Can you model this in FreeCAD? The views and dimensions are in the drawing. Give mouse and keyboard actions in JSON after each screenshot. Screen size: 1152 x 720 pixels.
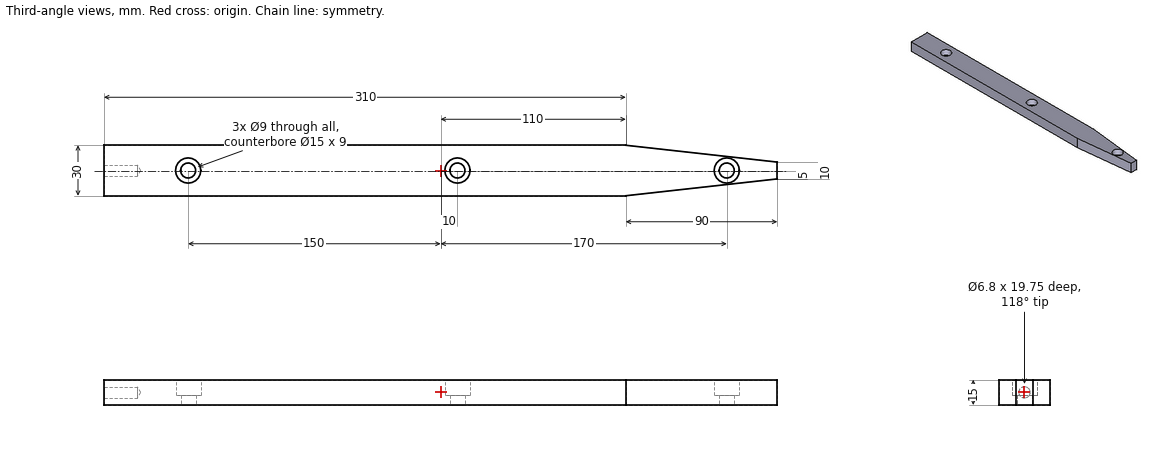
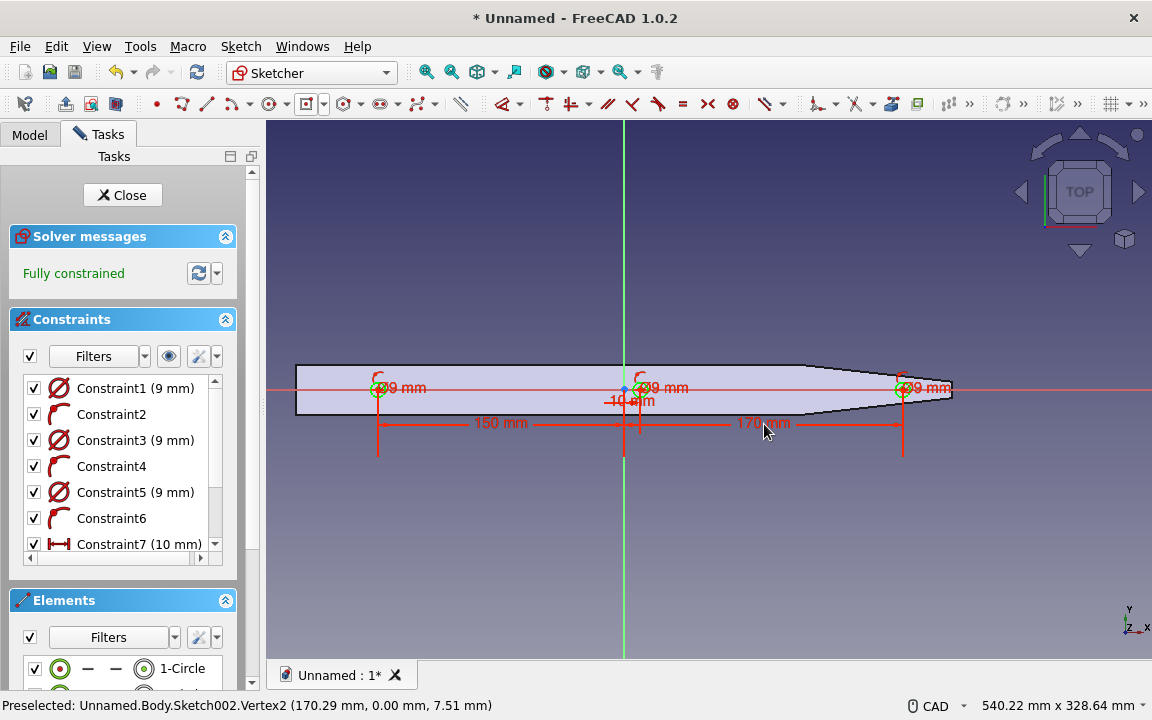
{"action": "left_click", "coordinate": [123, 195]}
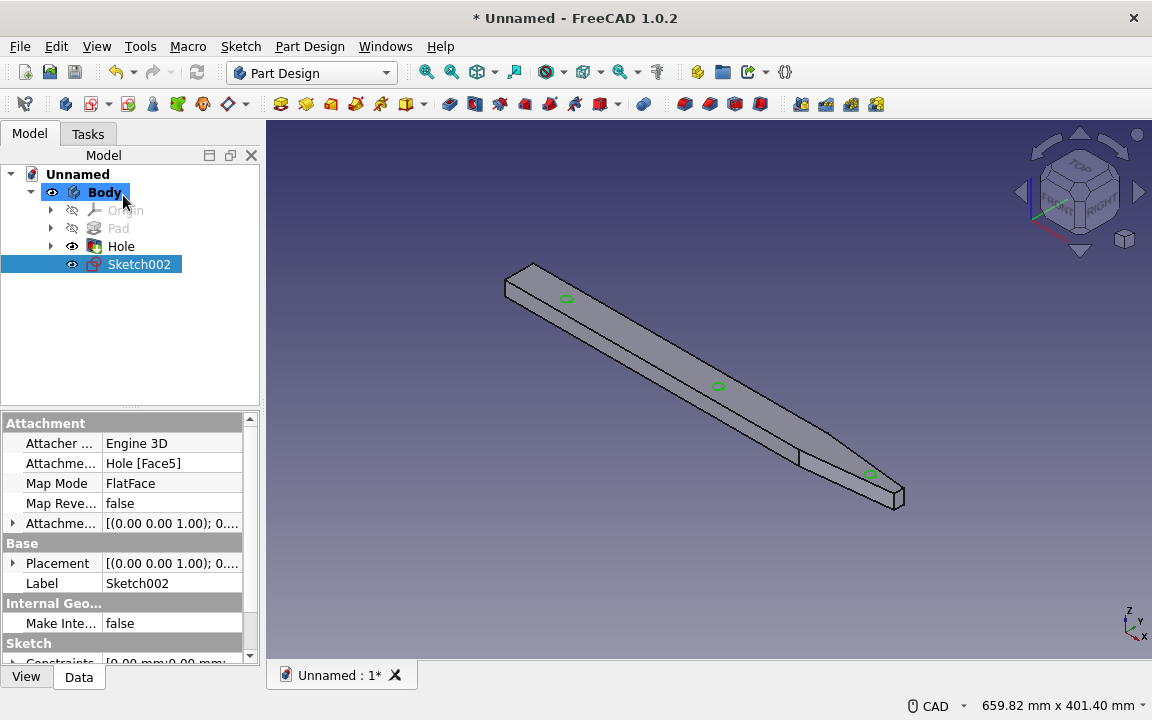
{"action": "left_click", "coordinate": [475, 104]}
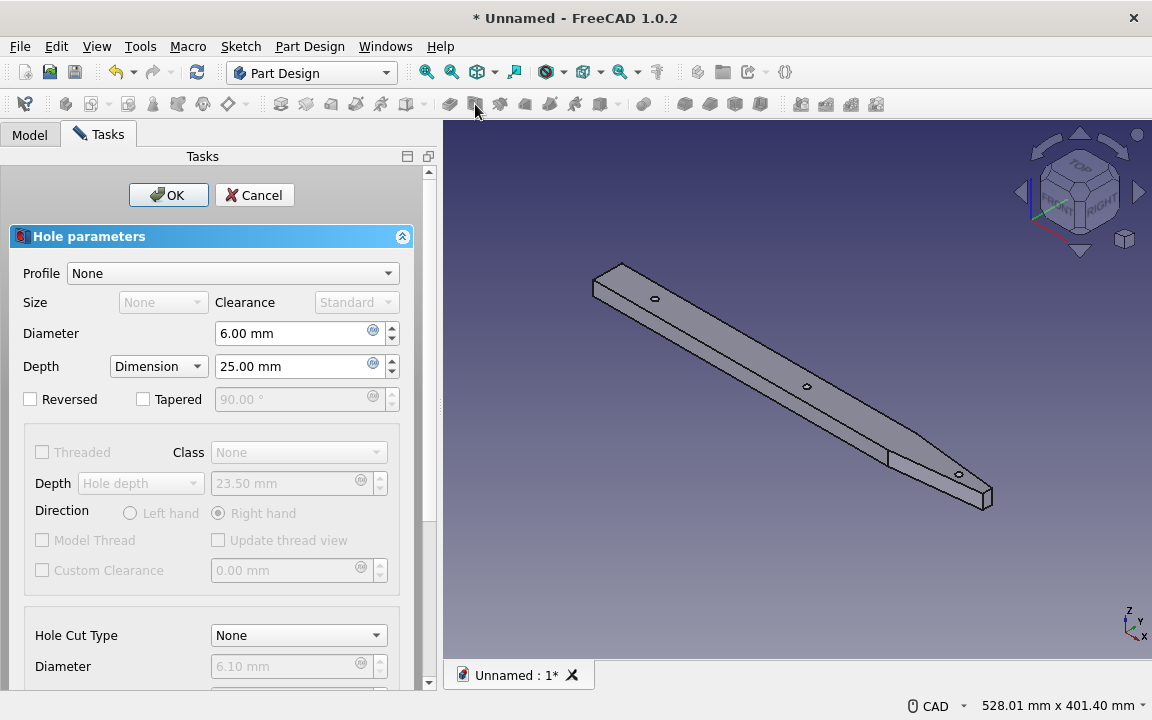
{"action": "triple_click", "coordinate": [300, 334]}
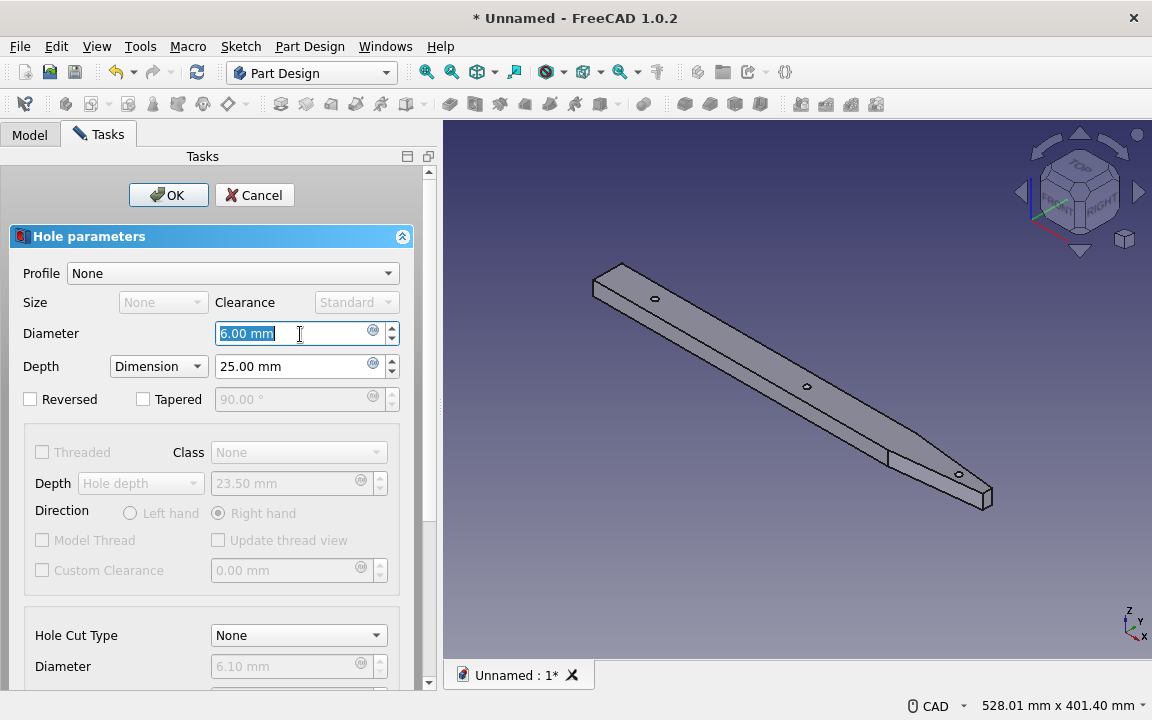
{"action": "type", "text": "9"}
{"action": "key", "text": "Tab"}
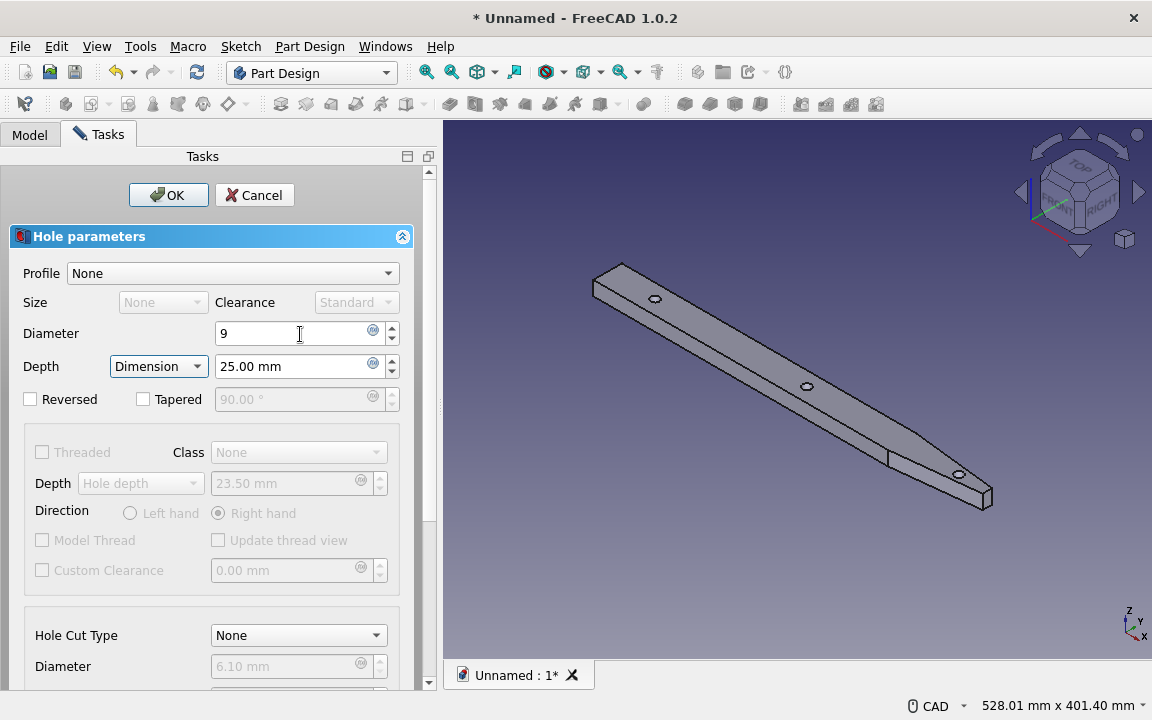
{"action": "left_click", "coordinate": [160, 366]}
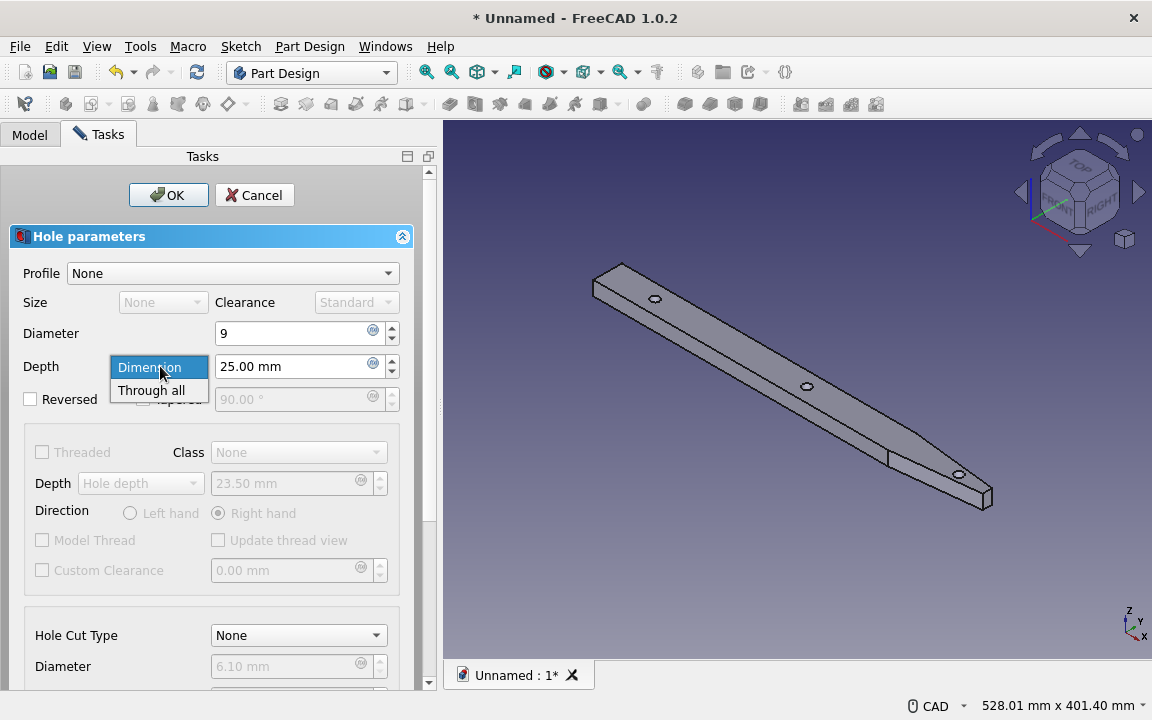
{"action": "left_click", "coordinate": [158, 390]}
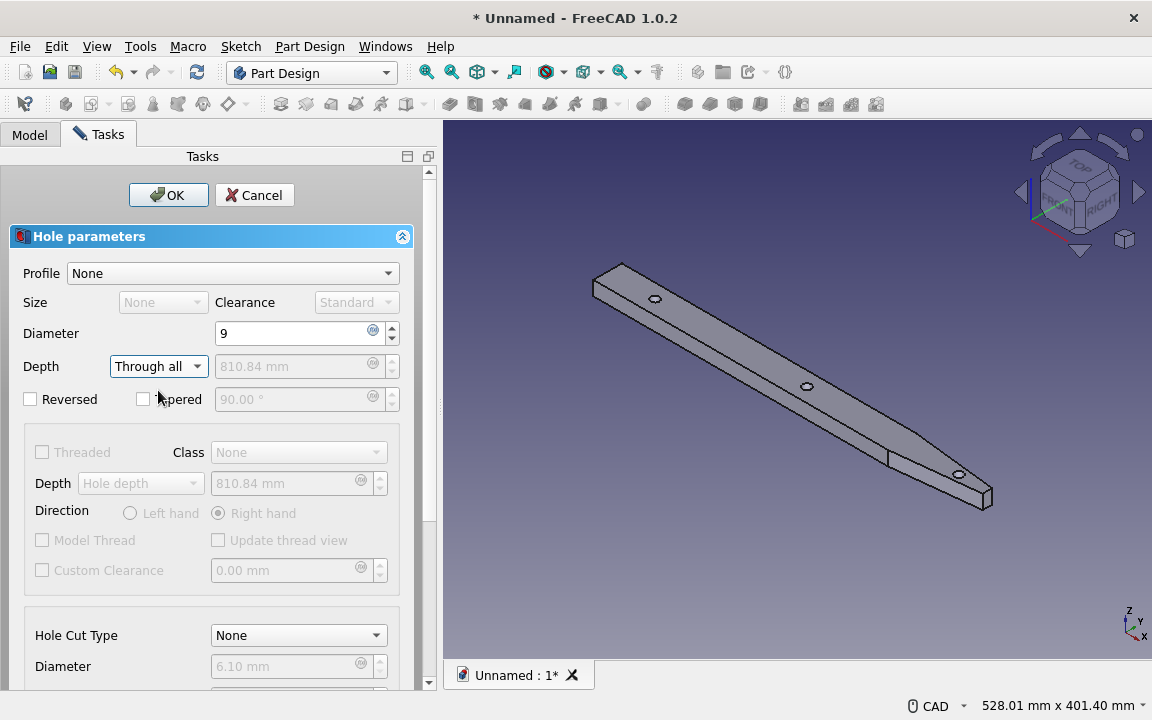
{"action": "left_click", "coordinate": [300, 636]}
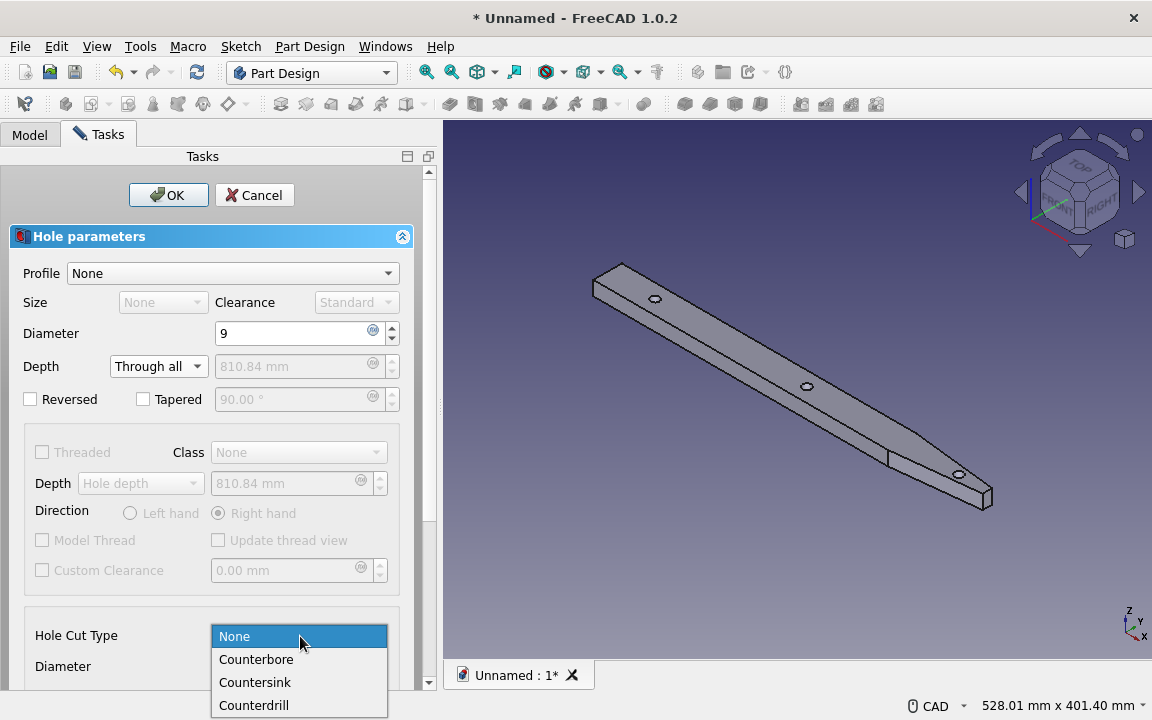
{"action": "left_click", "coordinate": [298, 660]}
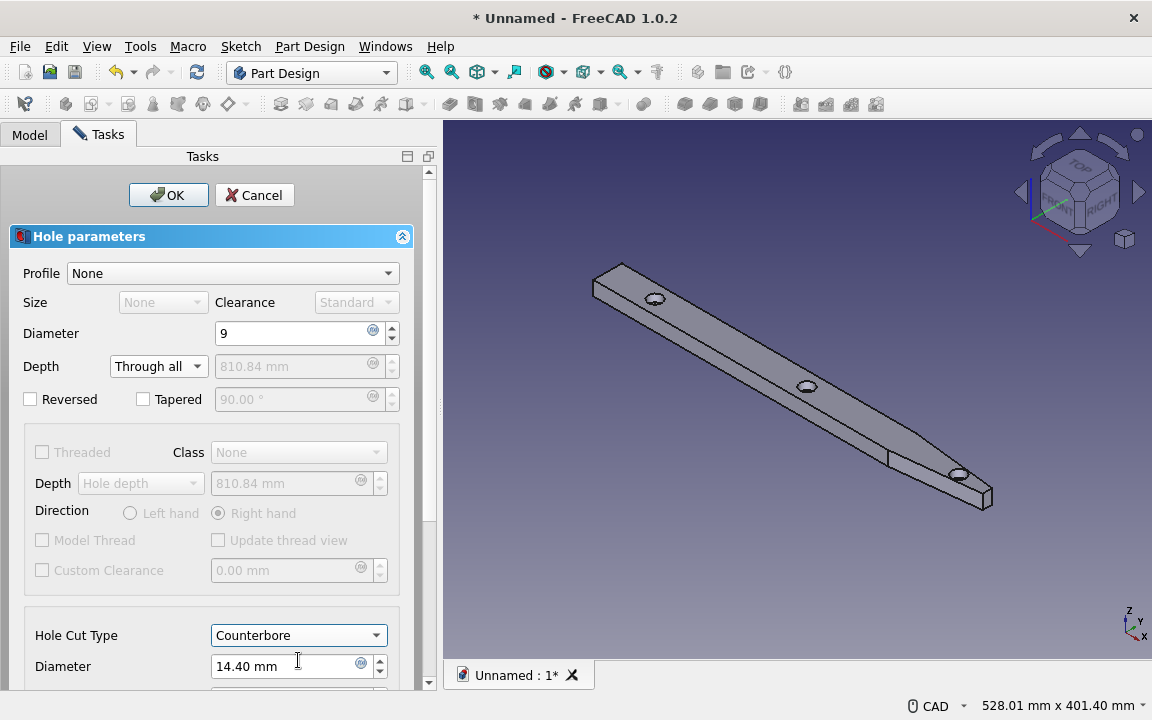
{"action": "triple_click", "coordinate": [292, 666]}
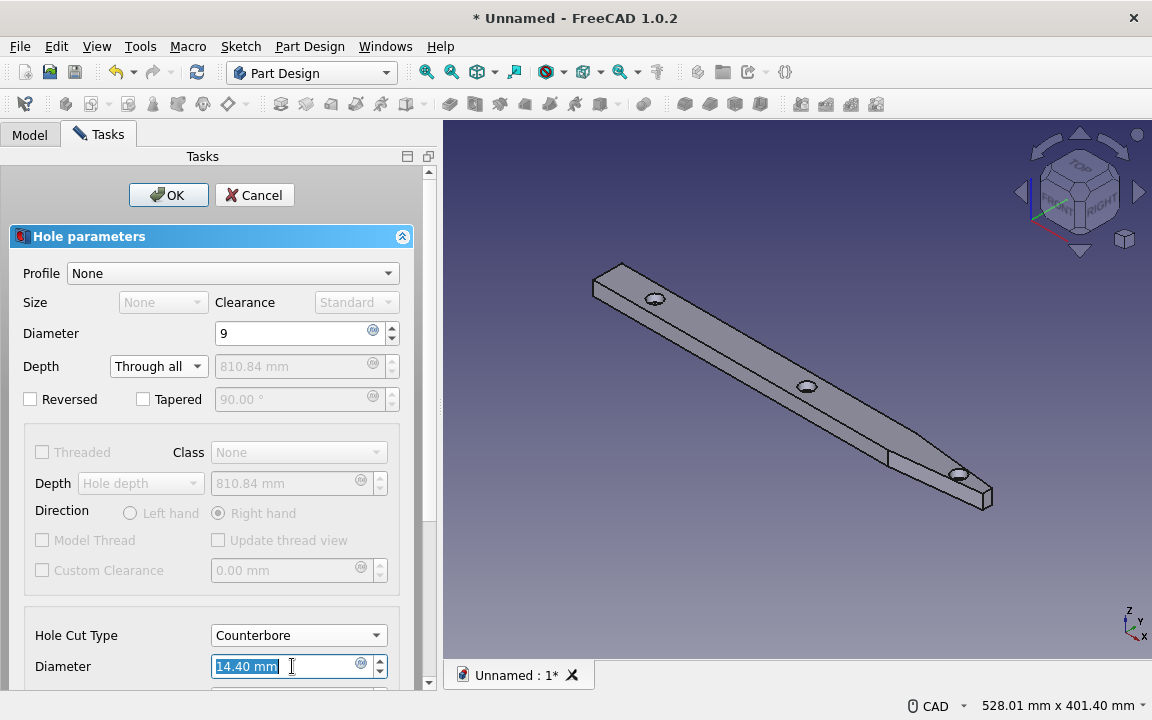
{"action": "type", "text": "15"}
{"action": "key", "text": "Tab"}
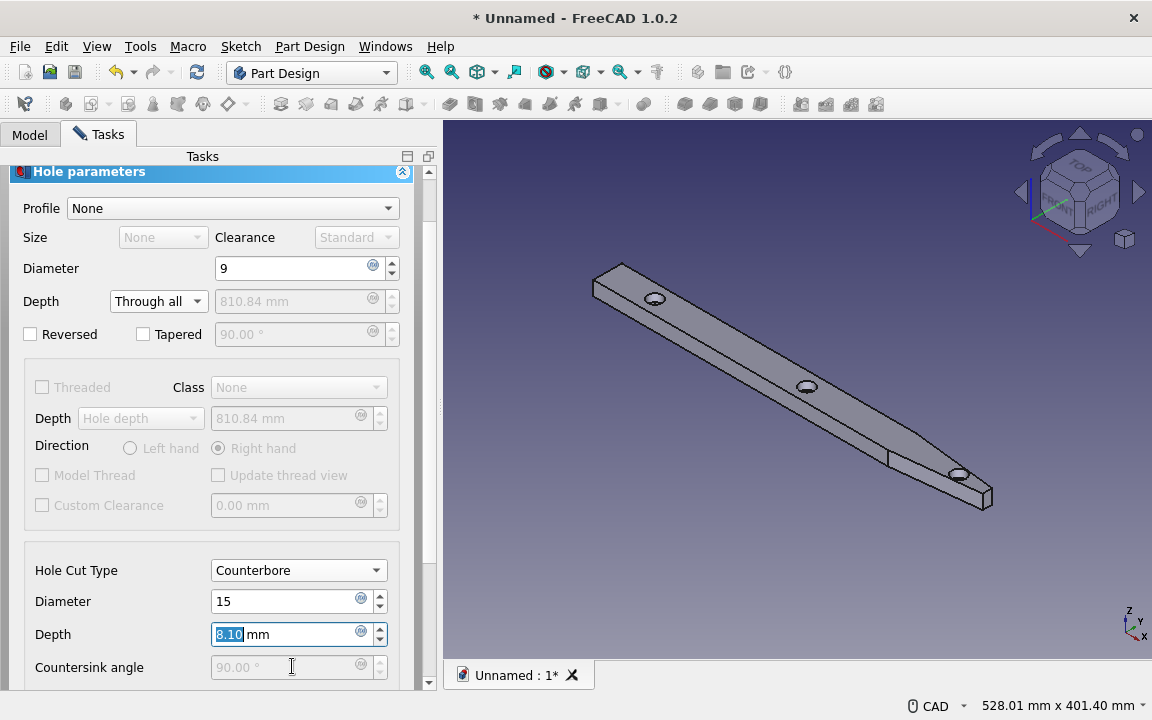
{"action": "type", "text": "9"}
{"action": "key", "text": "Tab"}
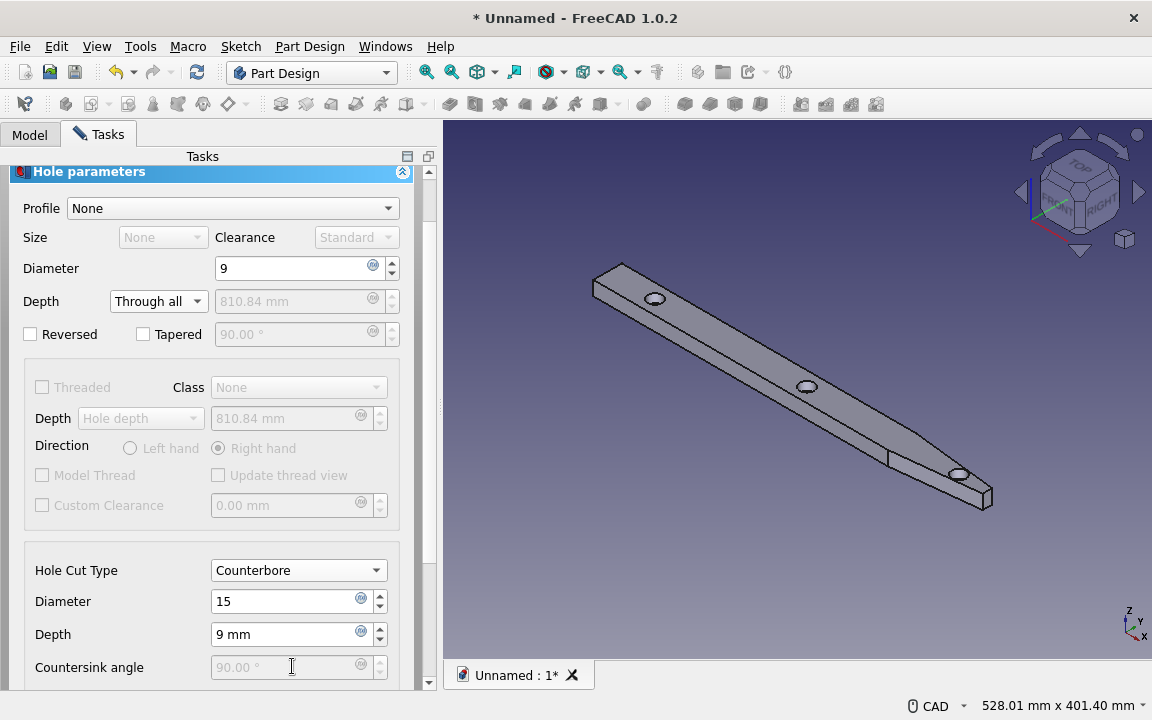
{"action": "scroll", "coordinate": [429, 428], "scroll_direction": "up", "scroll_amount": 2}